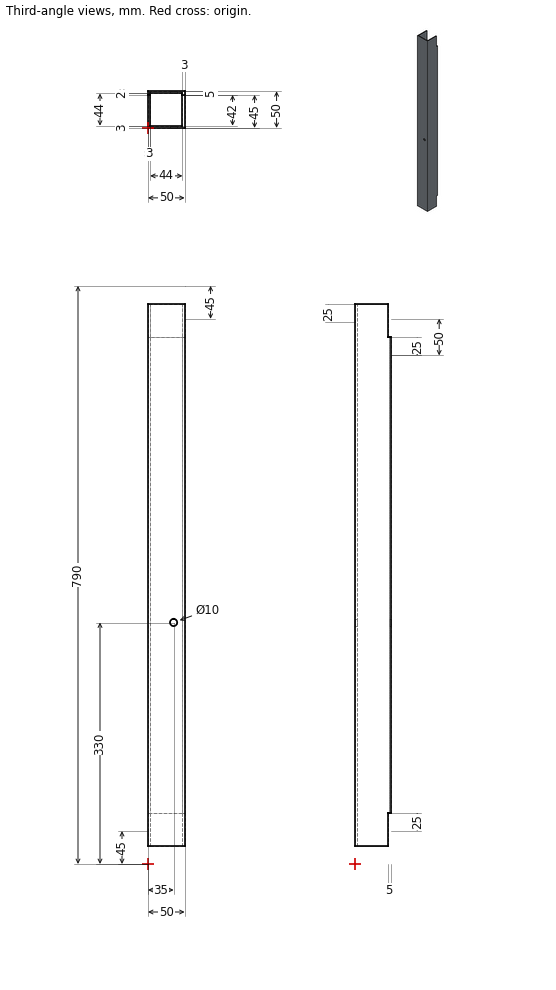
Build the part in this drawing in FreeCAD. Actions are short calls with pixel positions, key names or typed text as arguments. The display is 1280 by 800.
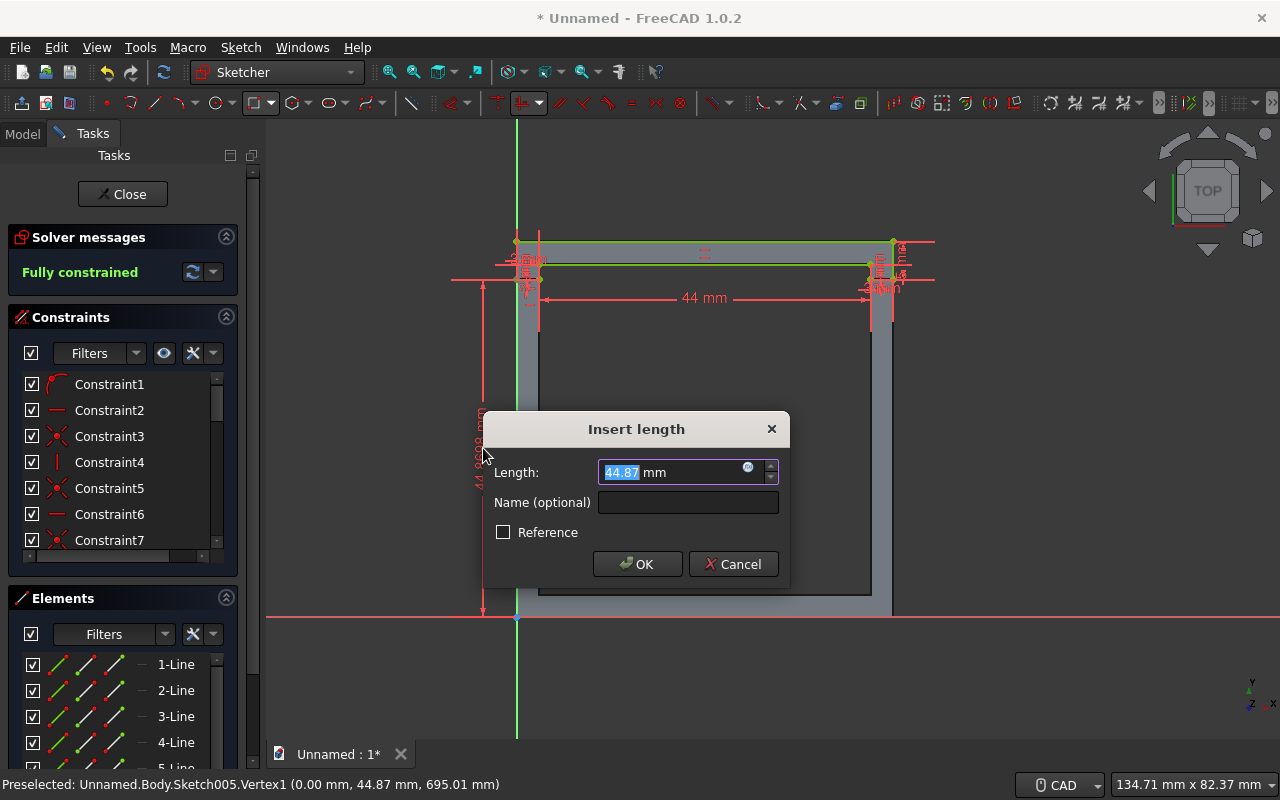
text(45)
key(Return)
key(Escape)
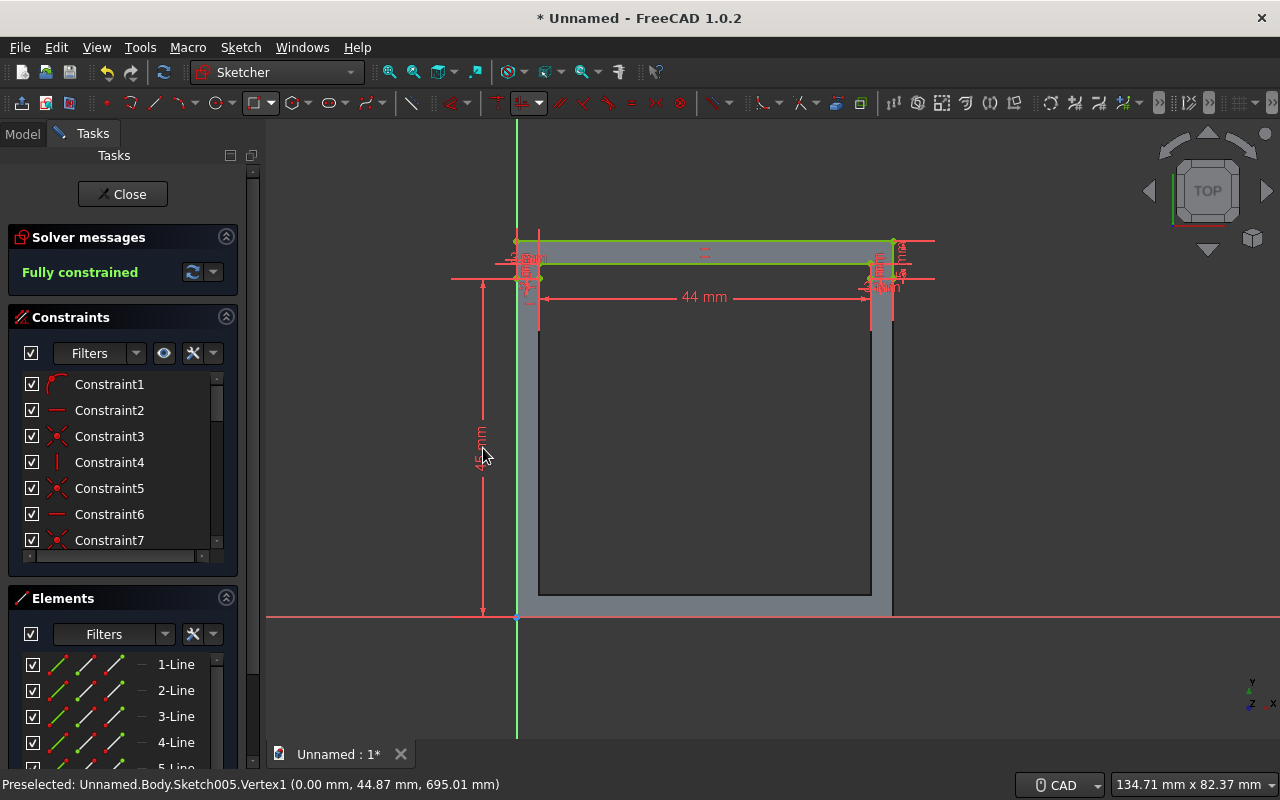
click(123, 194)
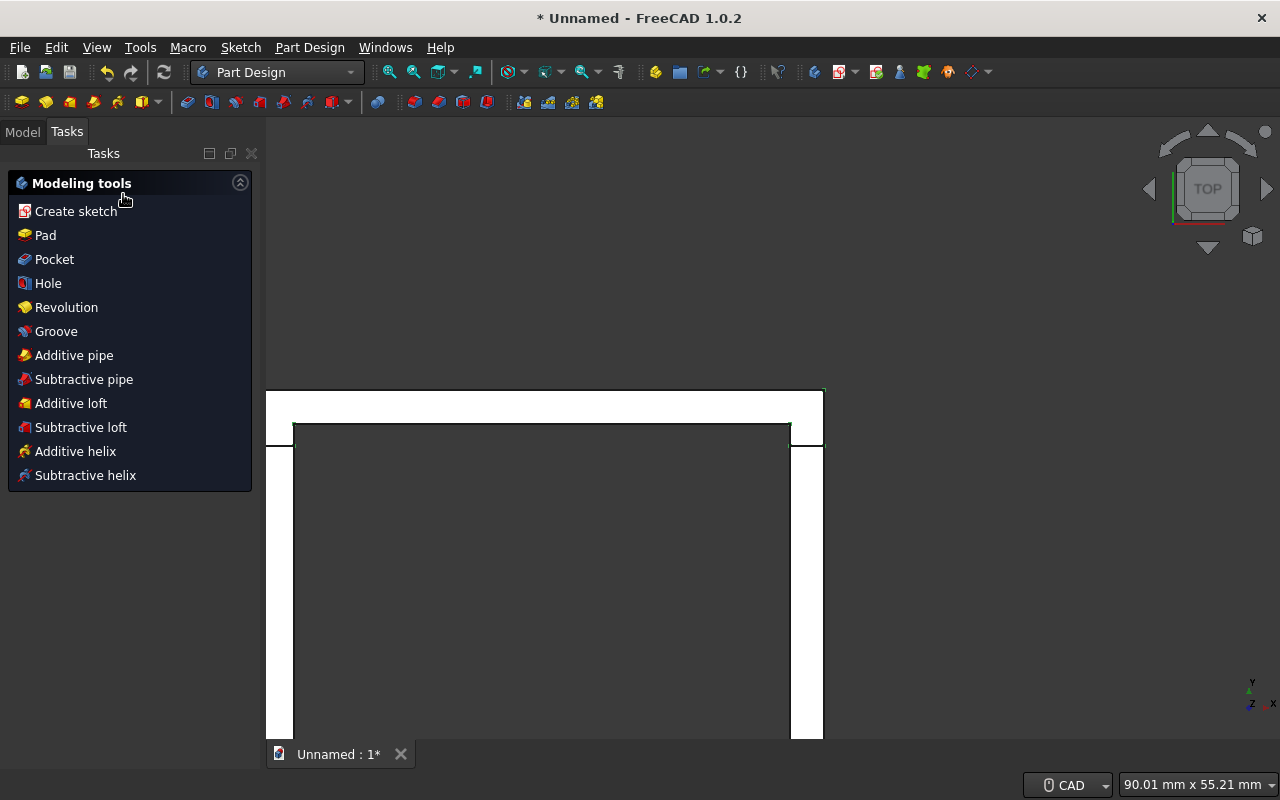
click(22, 102)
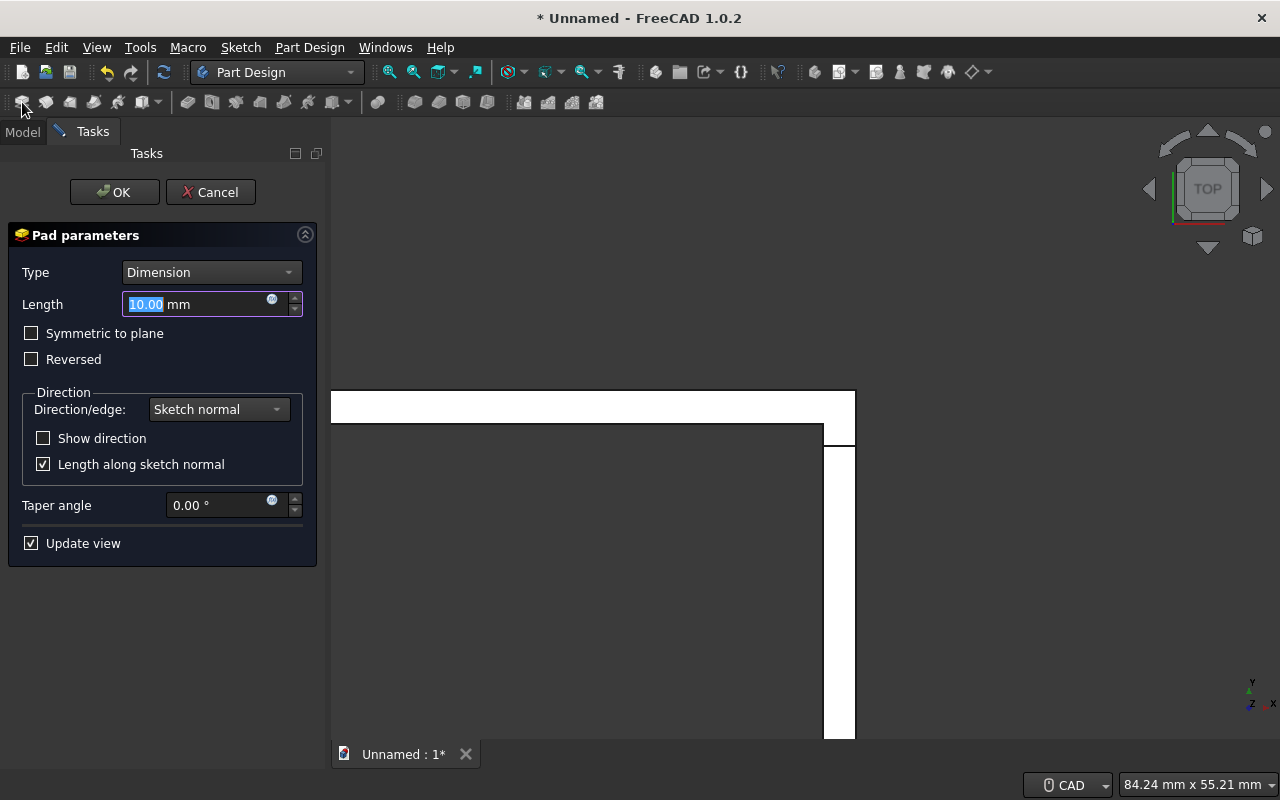
text(25)
key(Tab)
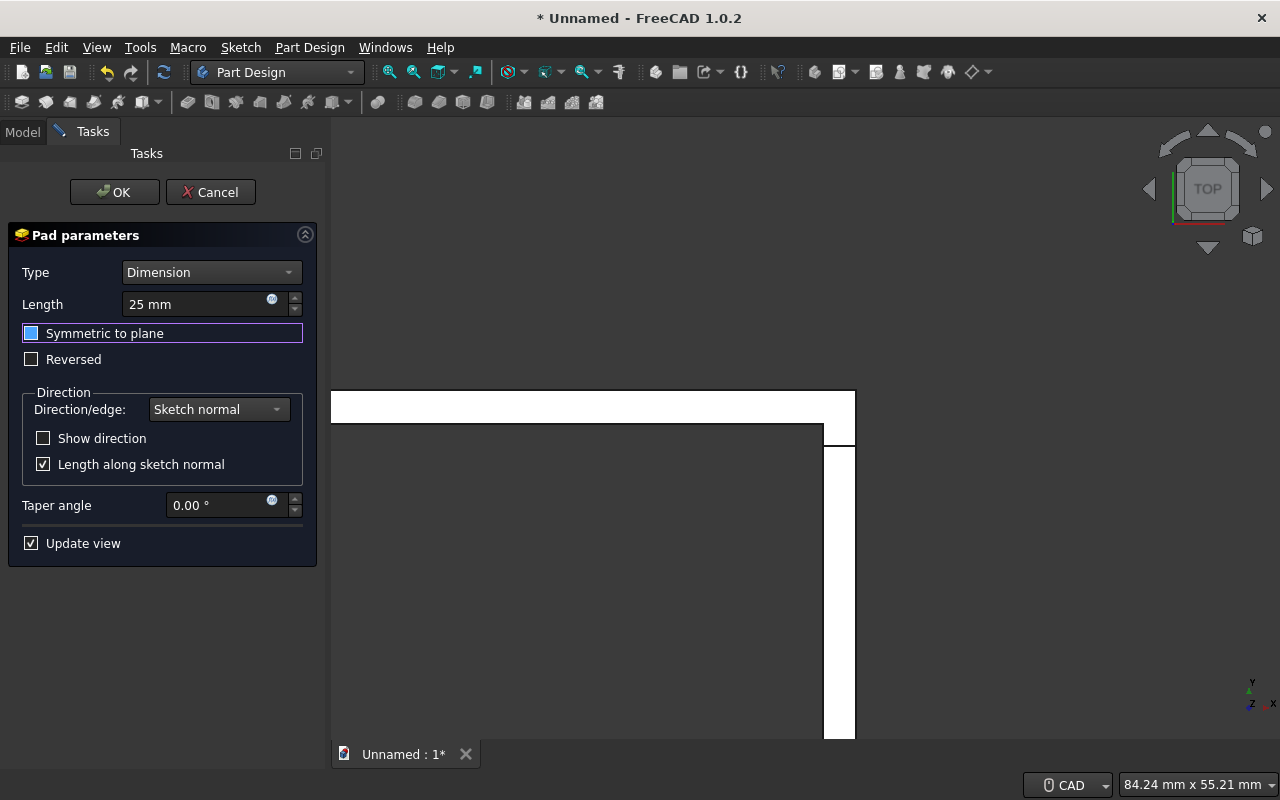
click(115, 192)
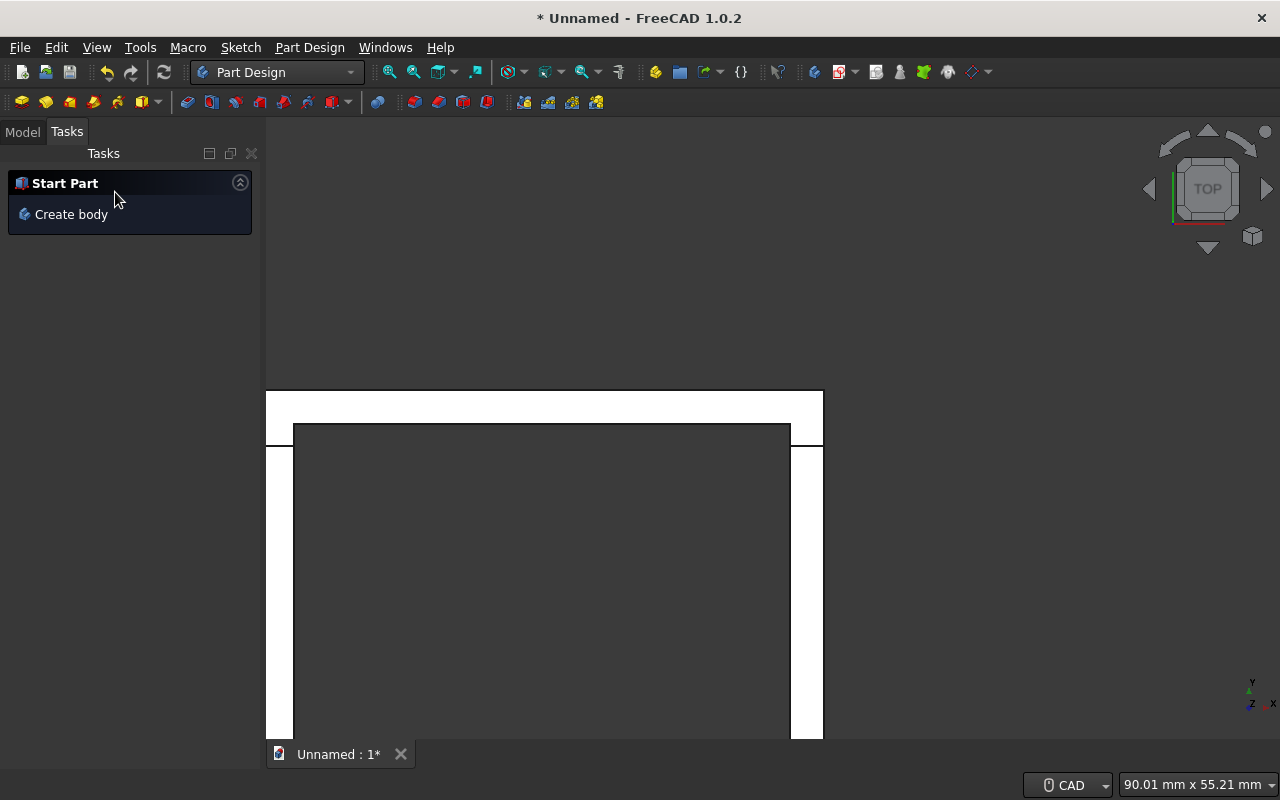
click(390, 72)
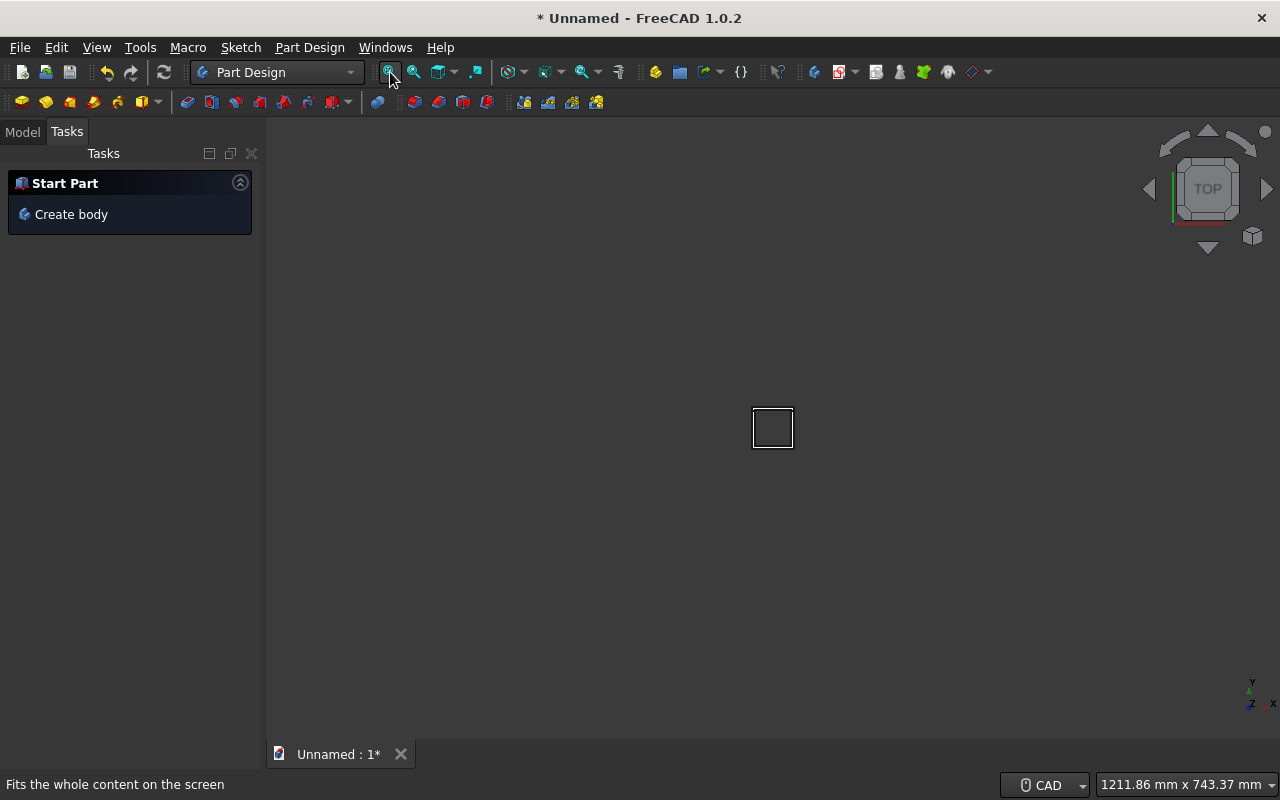
scroll(766, 446, up, 14)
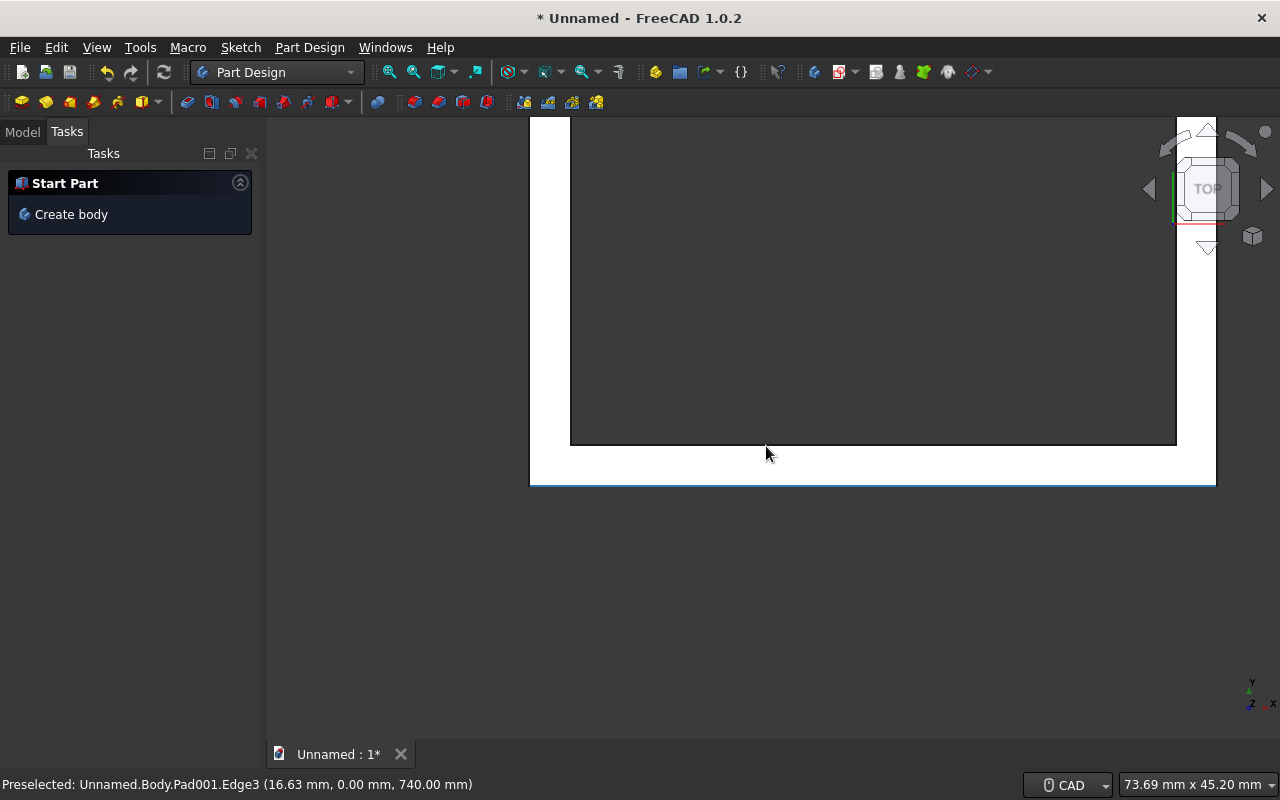
click(759, 457)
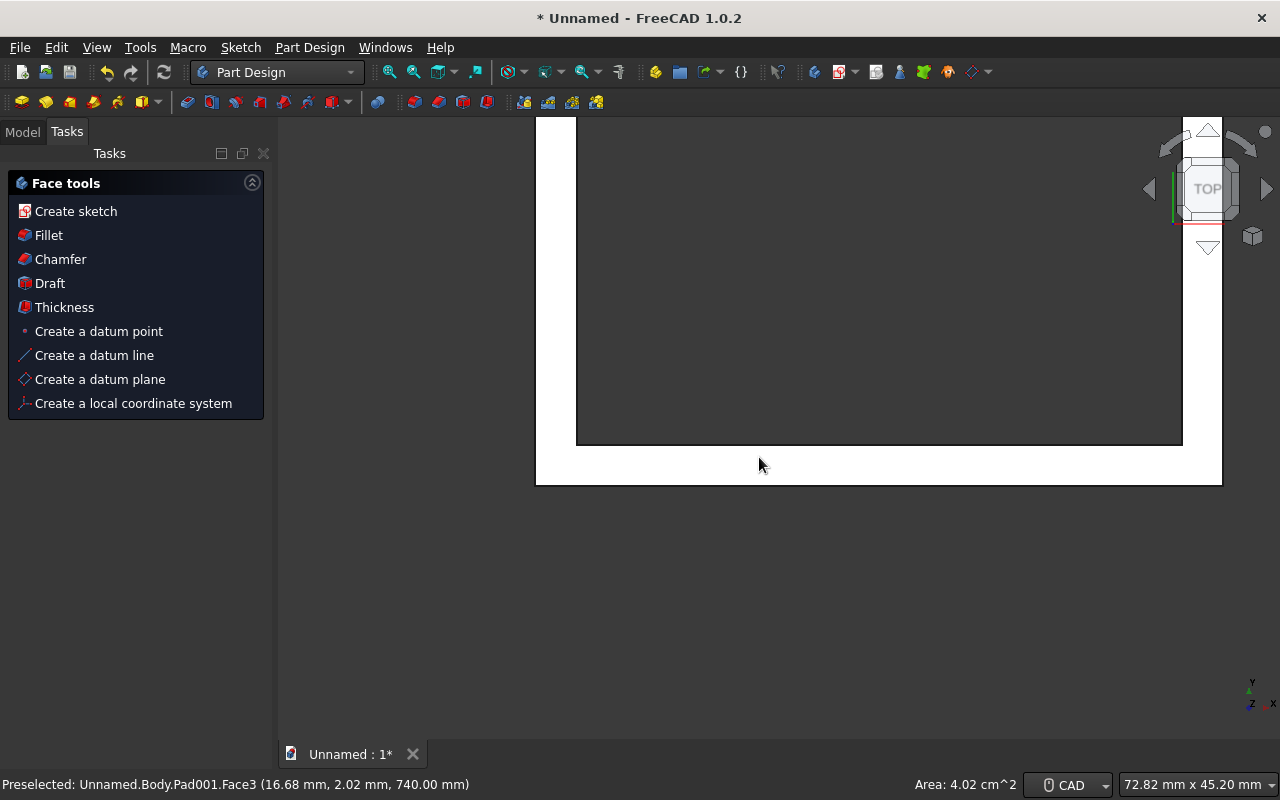
click(840, 72)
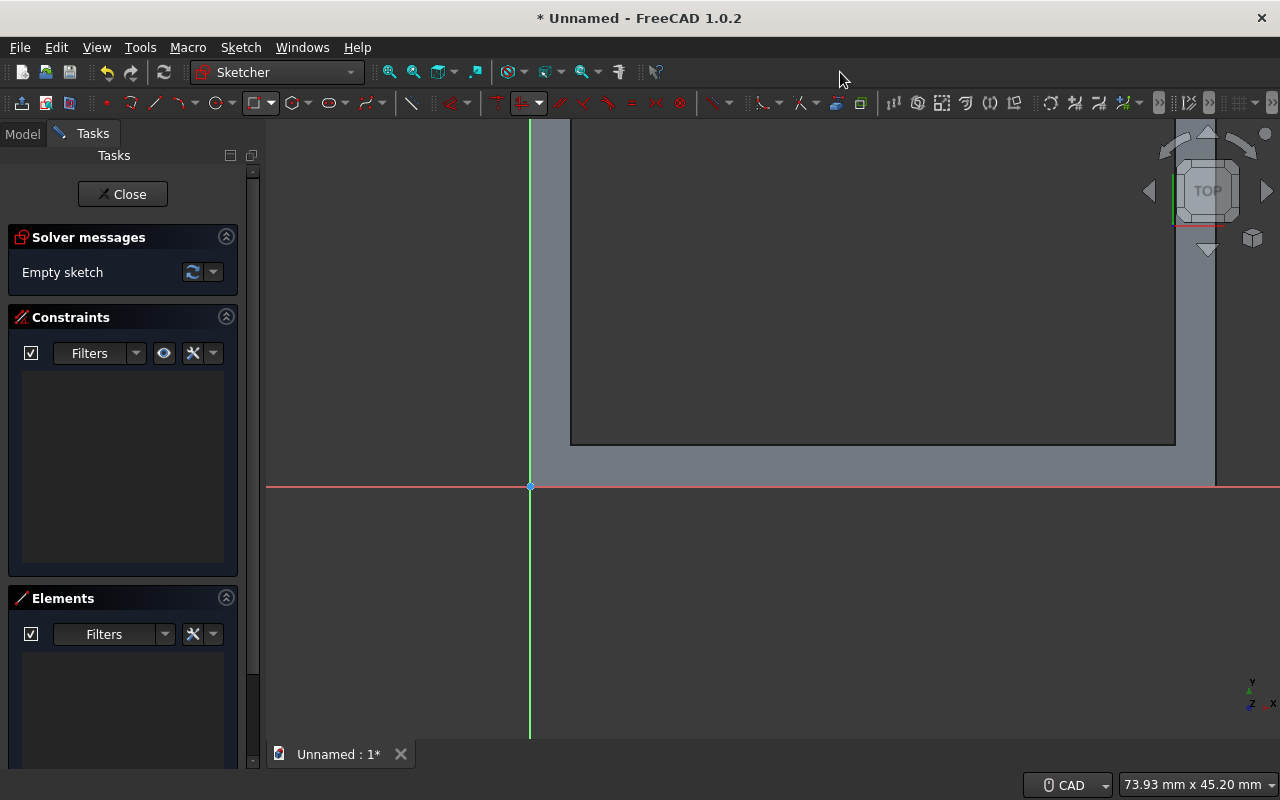
scroll(499, 711, down, 3)